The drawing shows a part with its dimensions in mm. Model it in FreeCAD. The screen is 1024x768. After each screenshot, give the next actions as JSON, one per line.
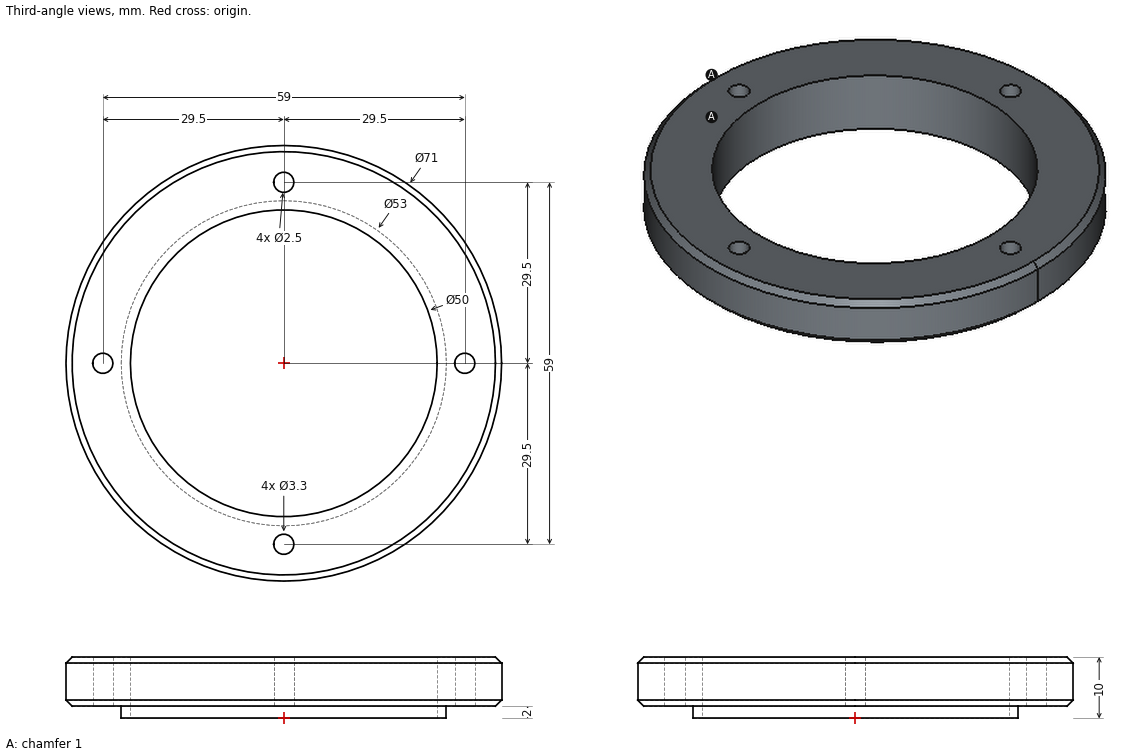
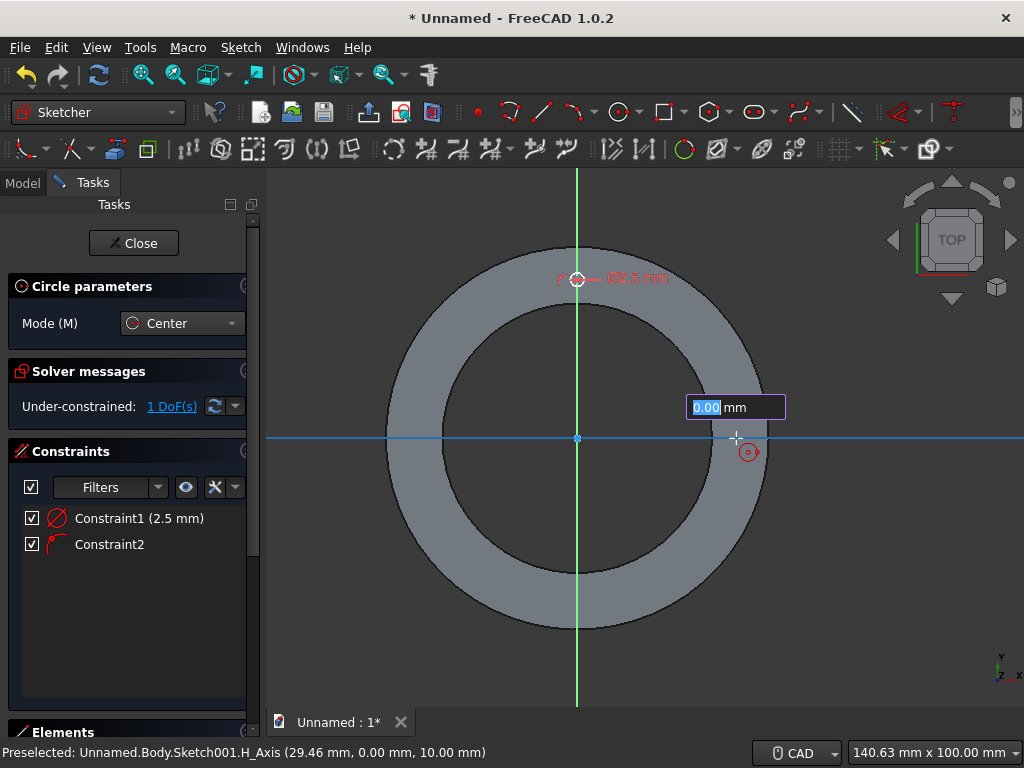
{"action": "scroll", "coordinate": [734, 445], "scroll_direction": "up", "scroll_amount": 5}
{"action": "mouse_move", "coordinate": [733, 443]}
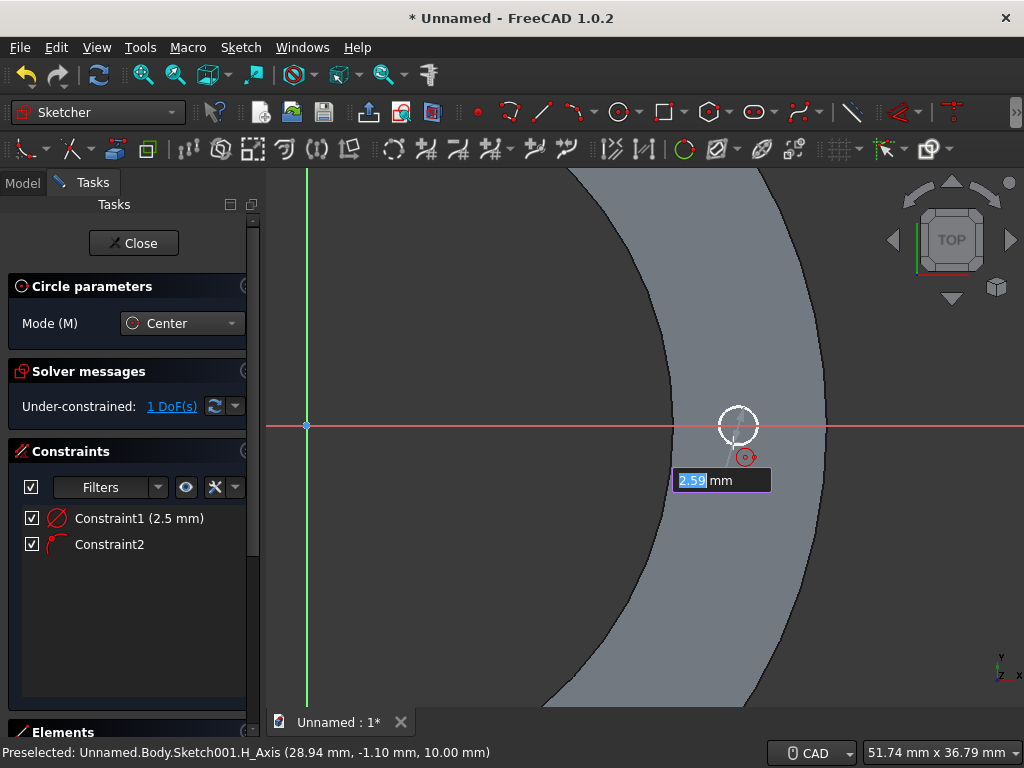
{"action": "type", "text": "2.5"}
{"action": "key", "text": "Return"}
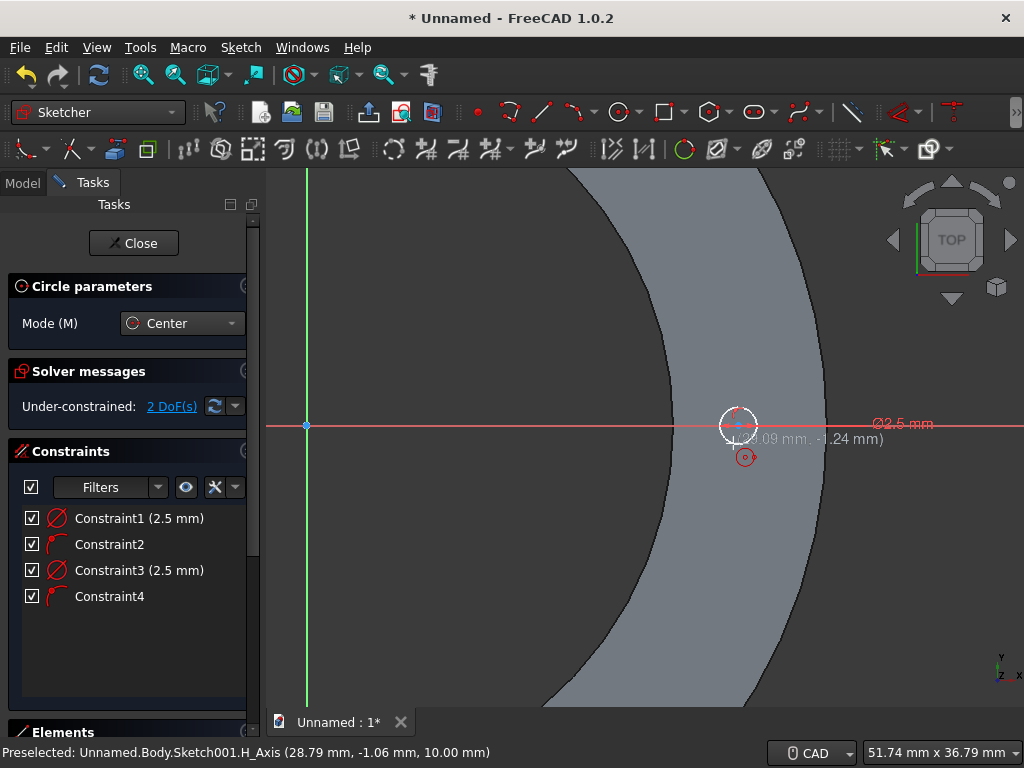
{"action": "scroll", "coordinate": [733, 444], "scroll_direction": "down", "scroll_amount": 5}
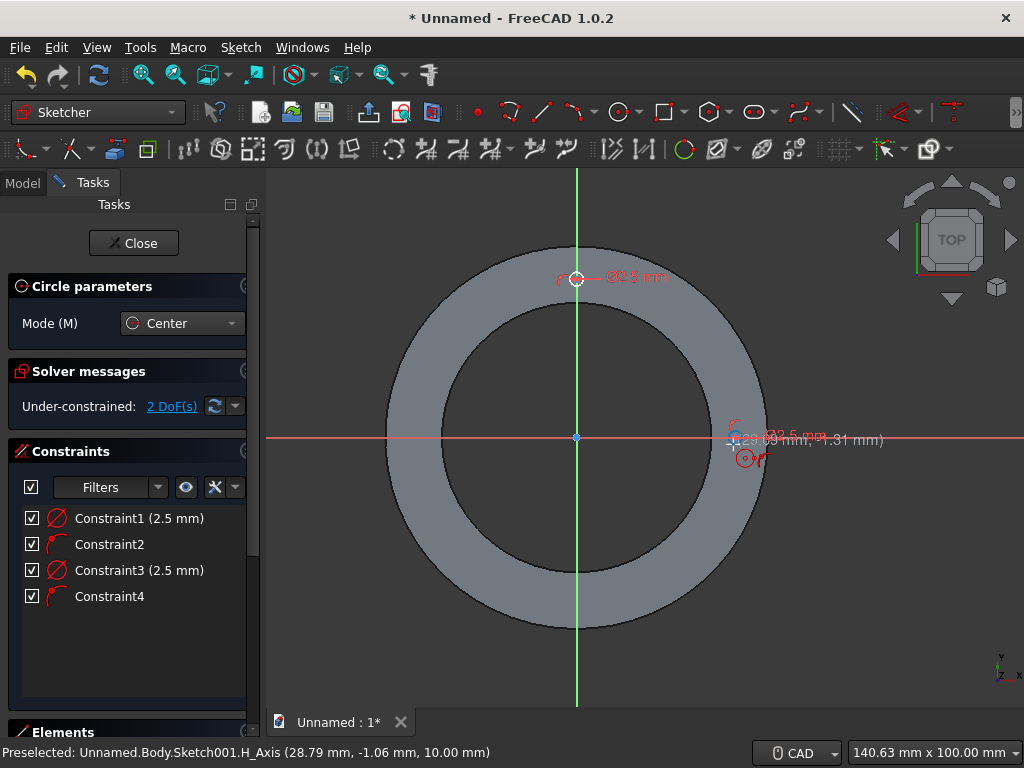
{"action": "scroll", "coordinate": [577, 597], "scroll_direction": "up", "scroll_amount": 7}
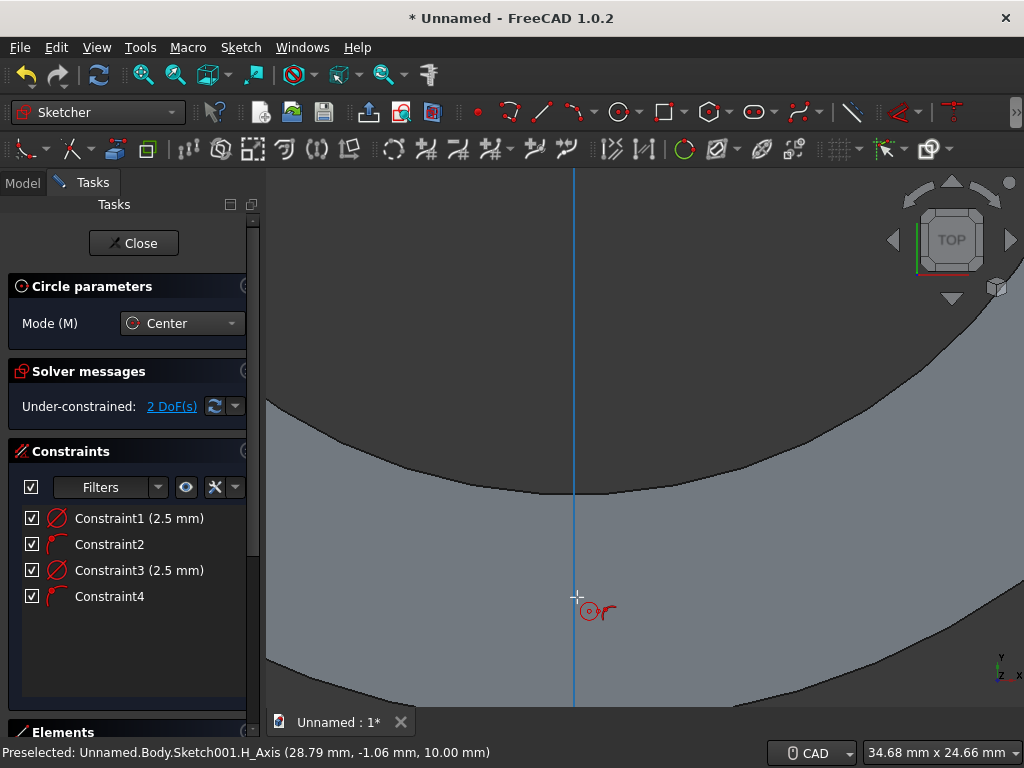
{"action": "scroll", "coordinate": [577, 598], "scroll_direction": "down", "scroll_amount": 7}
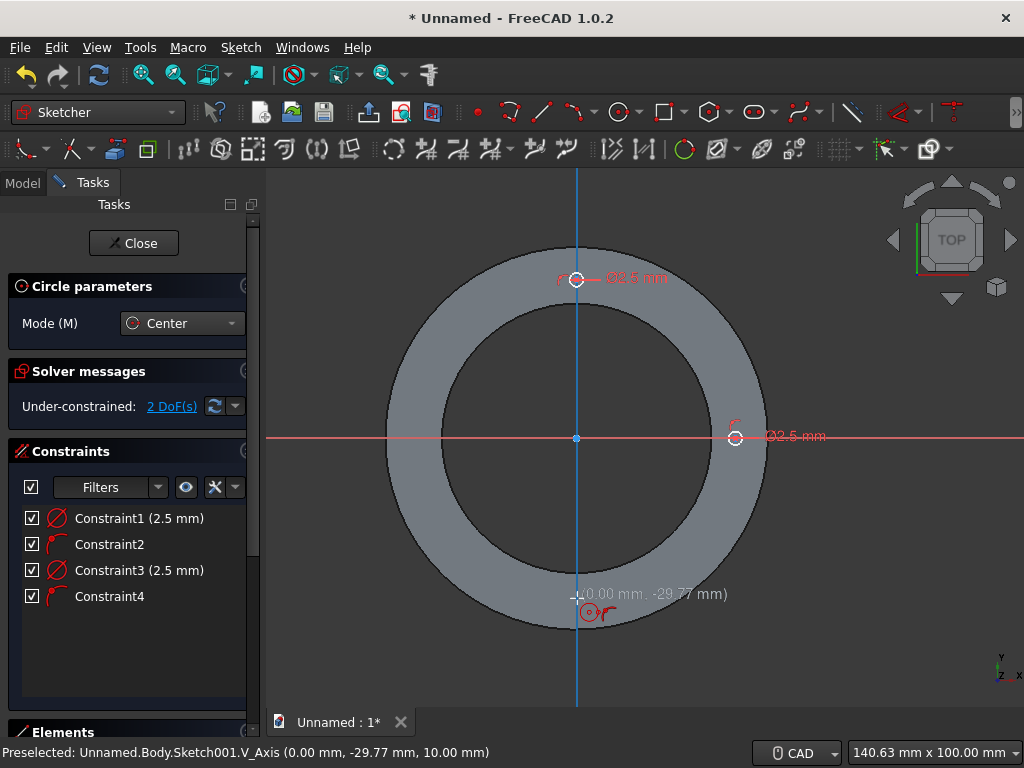
{"action": "left_click", "coordinate": [577, 597]}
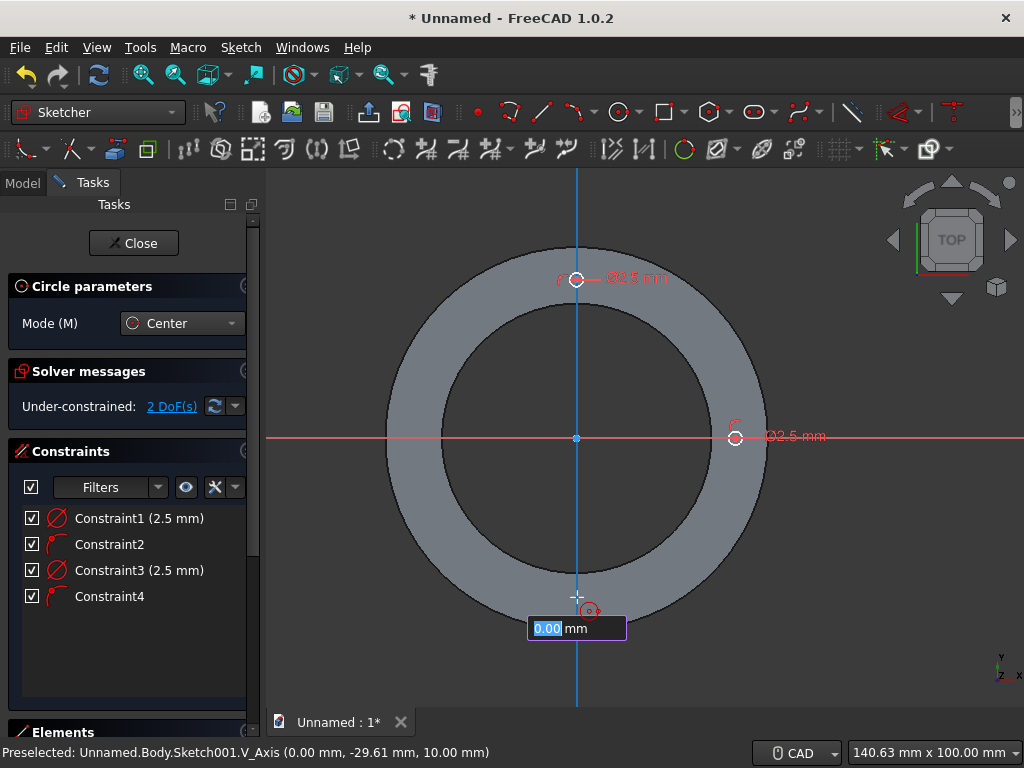
{"action": "scroll", "coordinate": [583, 595], "scroll_direction": "up", "scroll_amount": 5}
{"action": "mouse_move", "coordinate": [582, 594]}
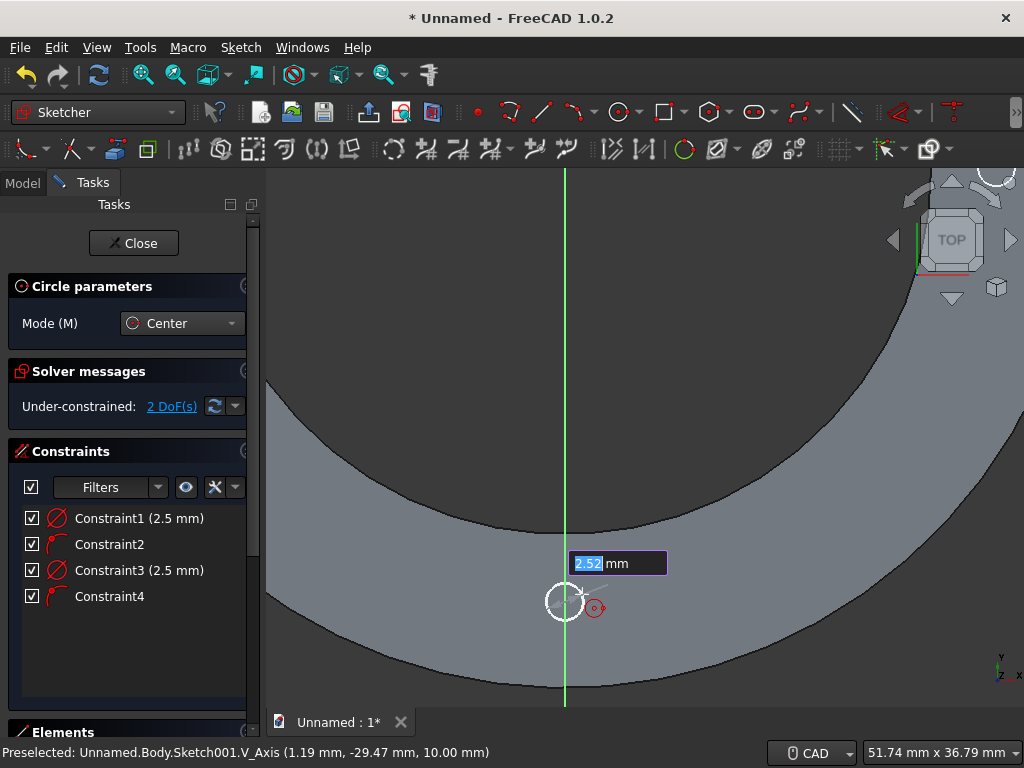
{"action": "type", "text": "2.5"}
{"action": "key", "text": "Return"}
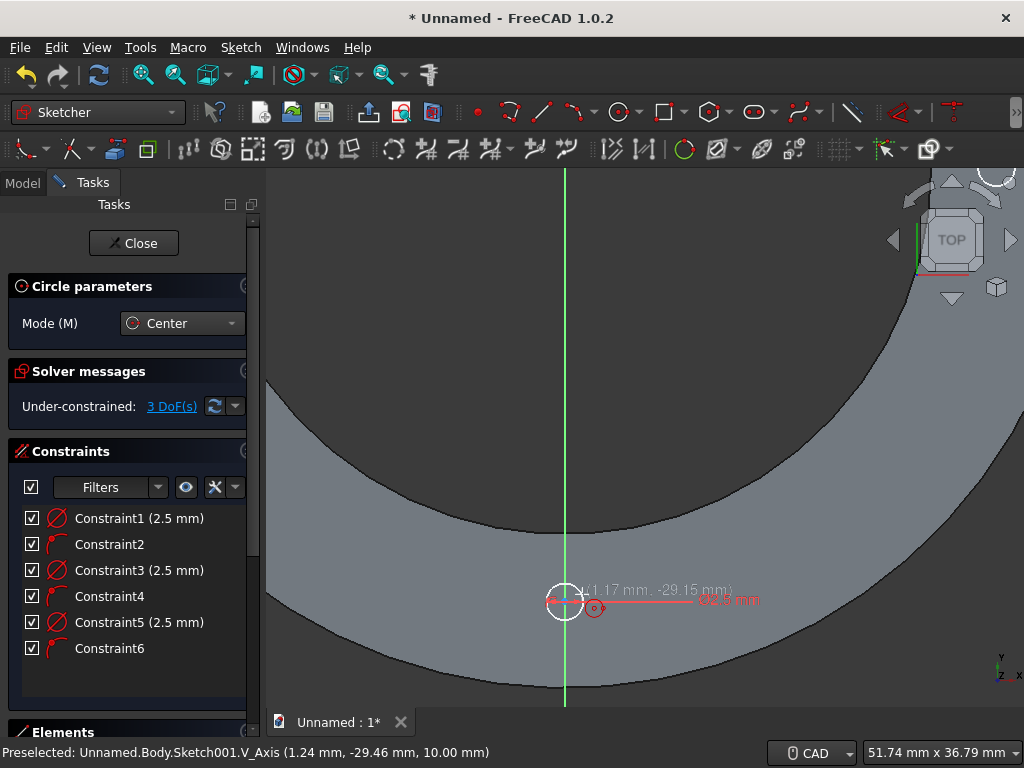
{"action": "scroll", "coordinate": [583, 594], "scroll_direction": "down", "scroll_amount": 5}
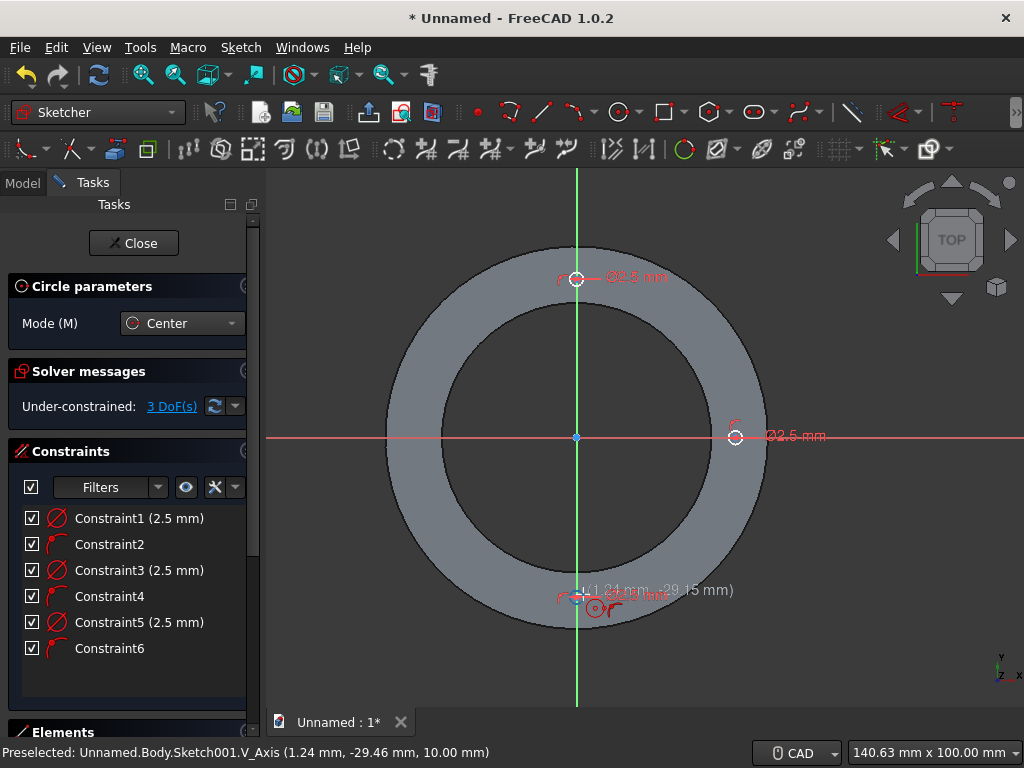
{"action": "scroll", "coordinate": [418, 438], "scroll_direction": "up", "scroll_amount": 7}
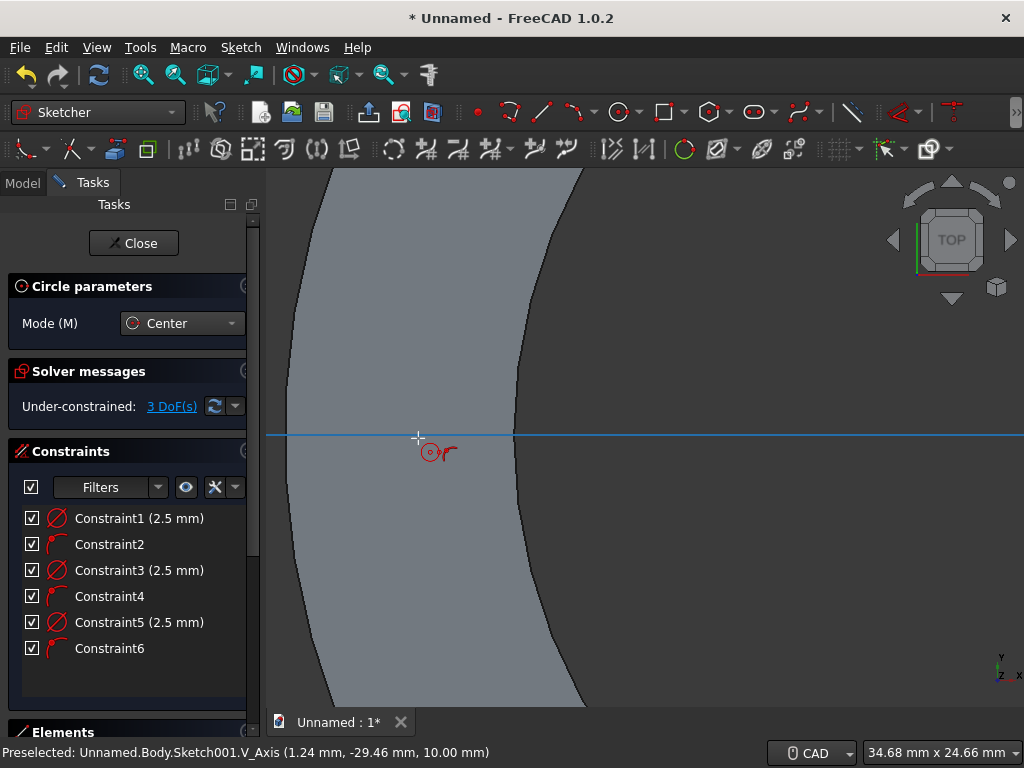
{"action": "scroll", "coordinate": [418, 438], "scroll_direction": "down", "scroll_amount": 7}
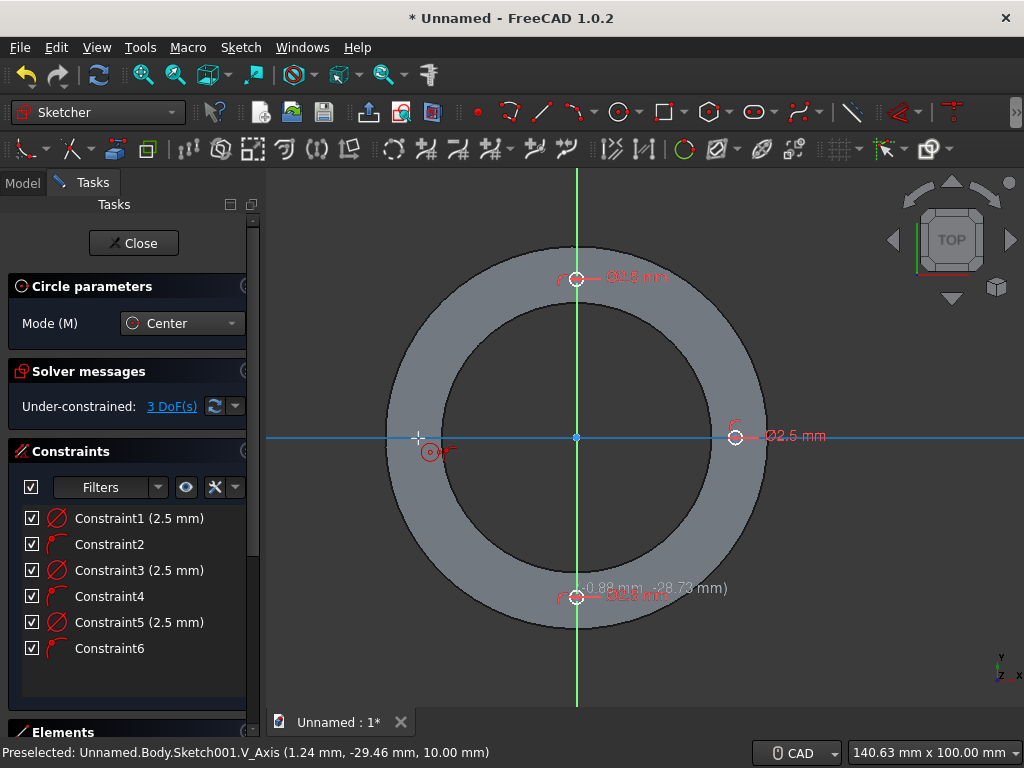
{"action": "left_click", "coordinate": [418, 438]}